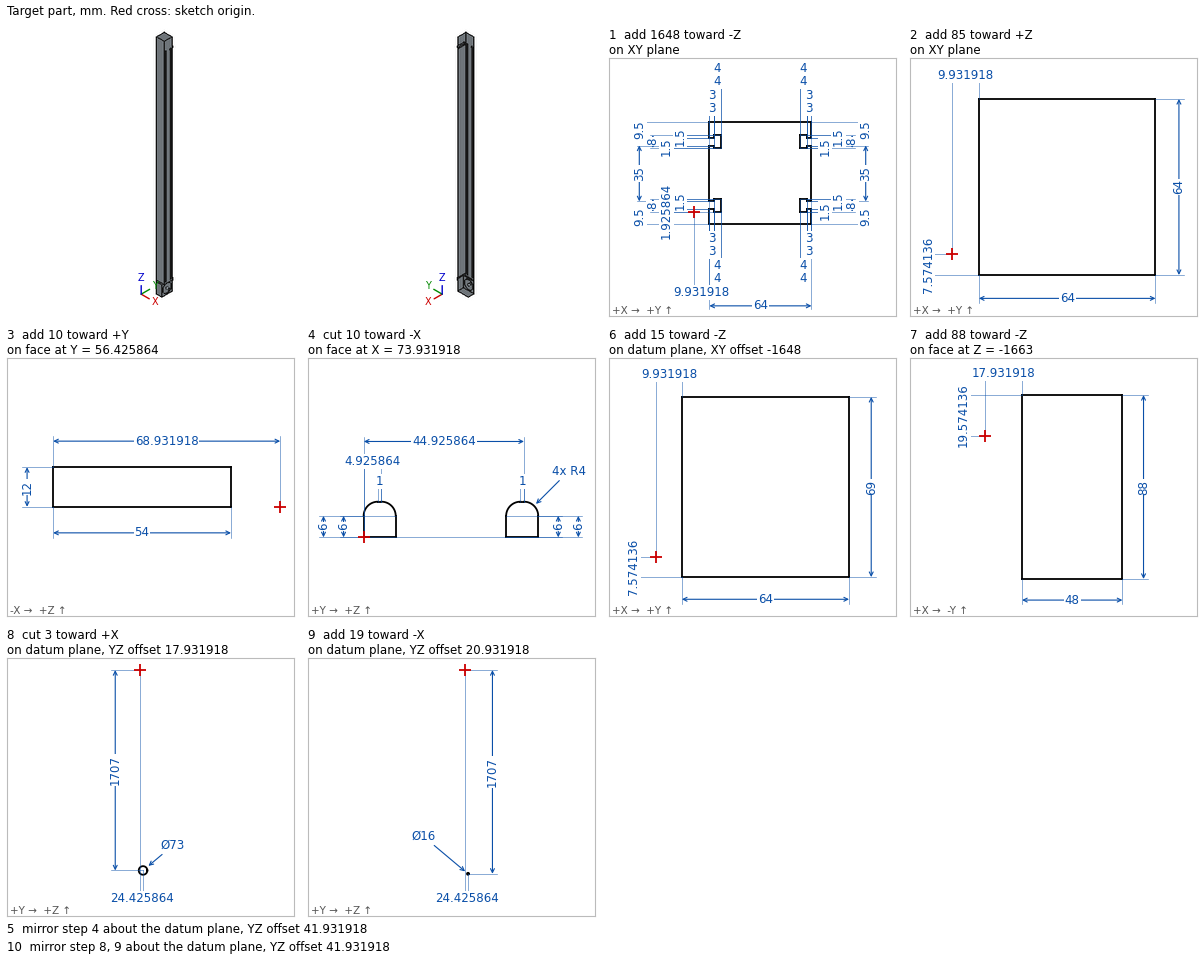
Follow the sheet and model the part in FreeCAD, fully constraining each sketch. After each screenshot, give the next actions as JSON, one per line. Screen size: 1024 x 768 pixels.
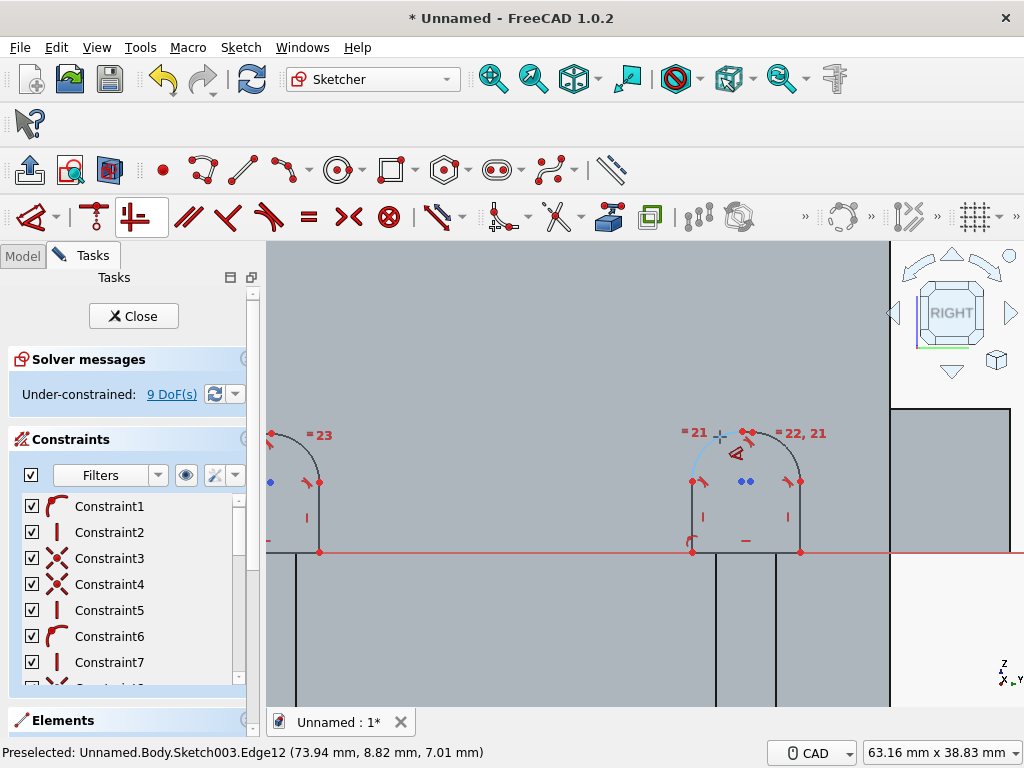
{"action": "left_click", "coordinate": [720, 437]}
{"action": "left_click", "coordinate": [706, 408]}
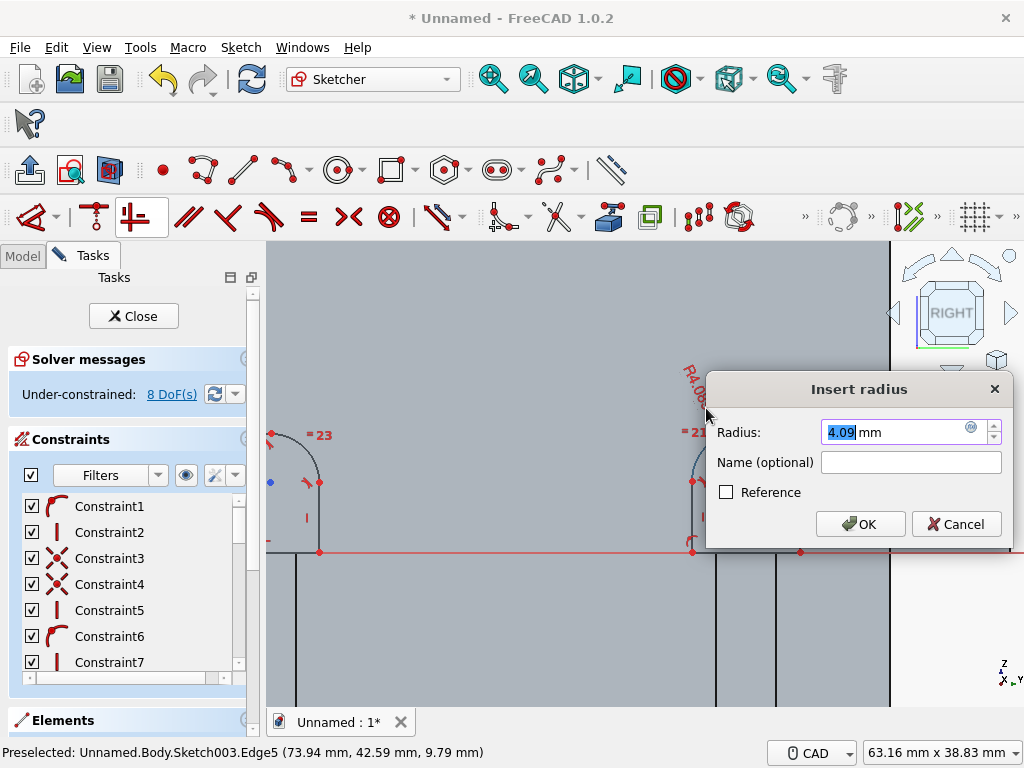
{"action": "type", "text": "4"}
{"action": "key", "text": "Return"}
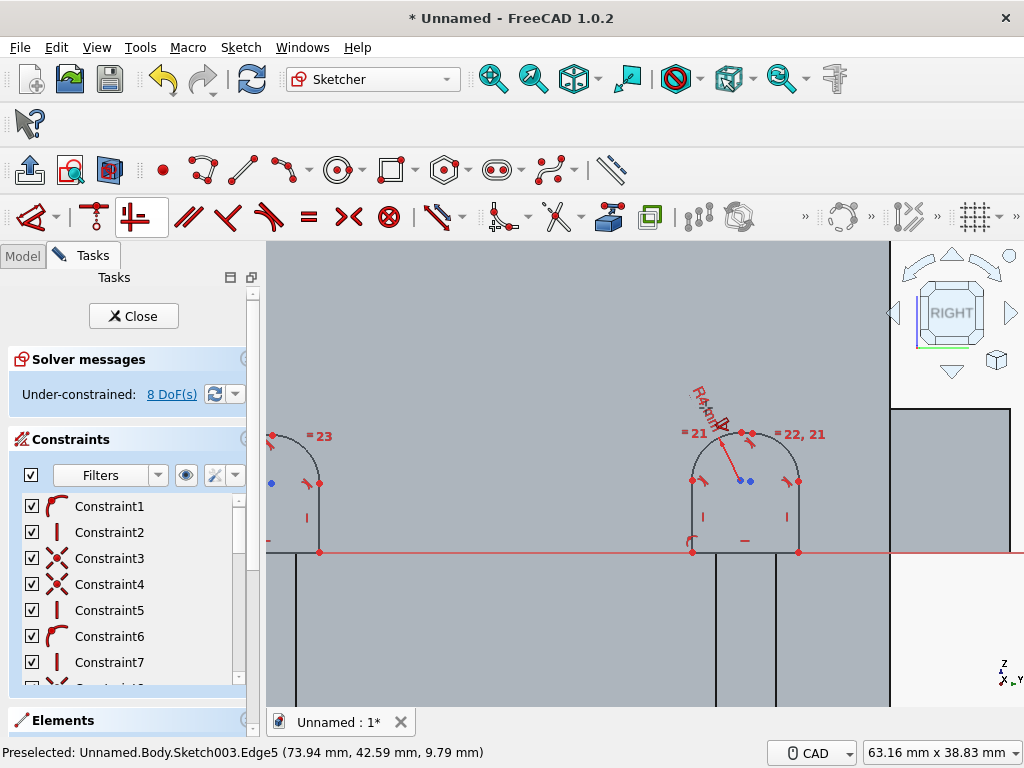
{"action": "scroll", "coordinate": [747, 433], "scroll_direction": "up", "scroll_amount": 6}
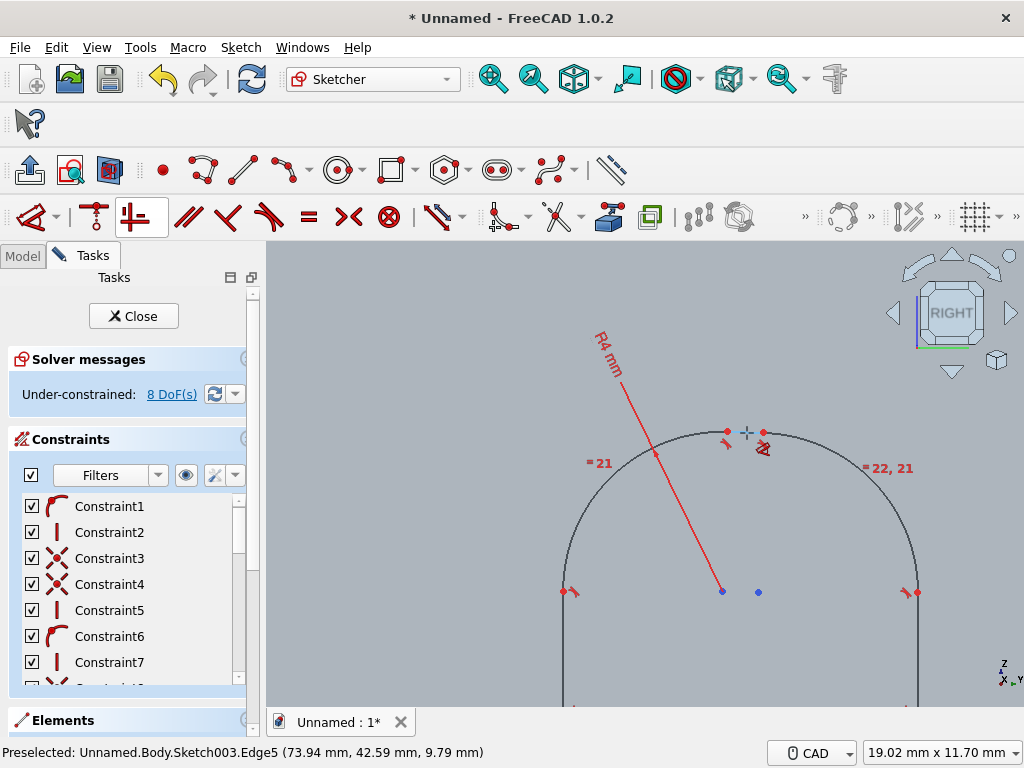
{"action": "left_click", "coordinate": [745, 432]}
{"action": "left_click", "coordinate": [745, 398]}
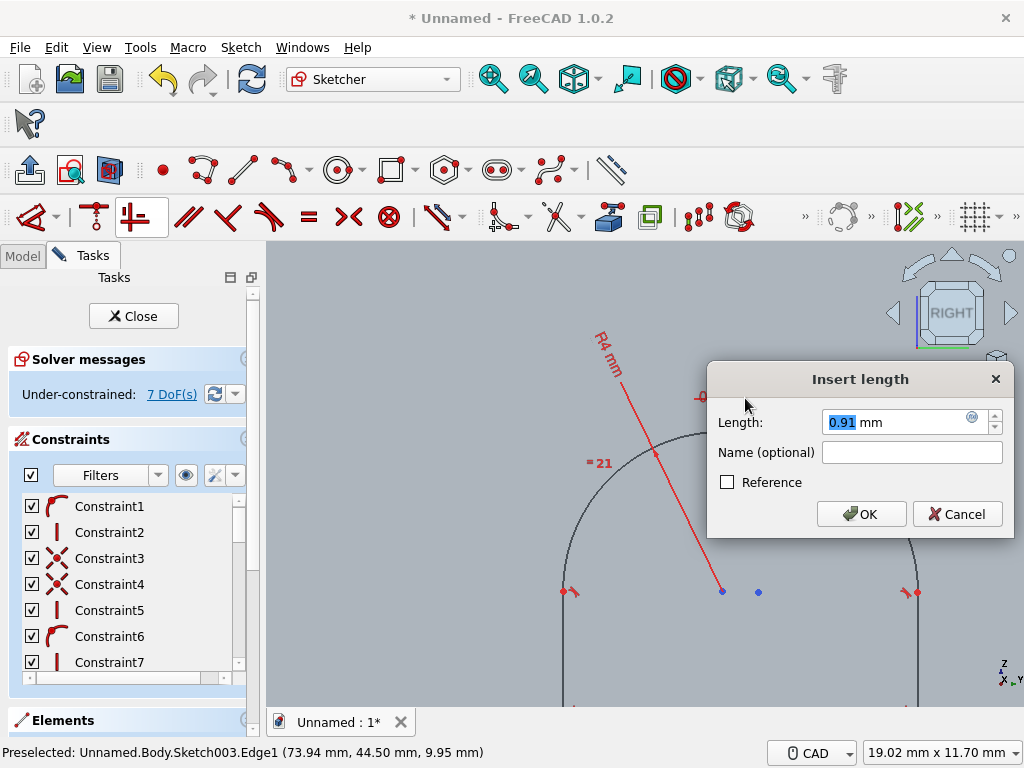
{"action": "type", "text": "1"}
{"action": "key", "text": "Return"}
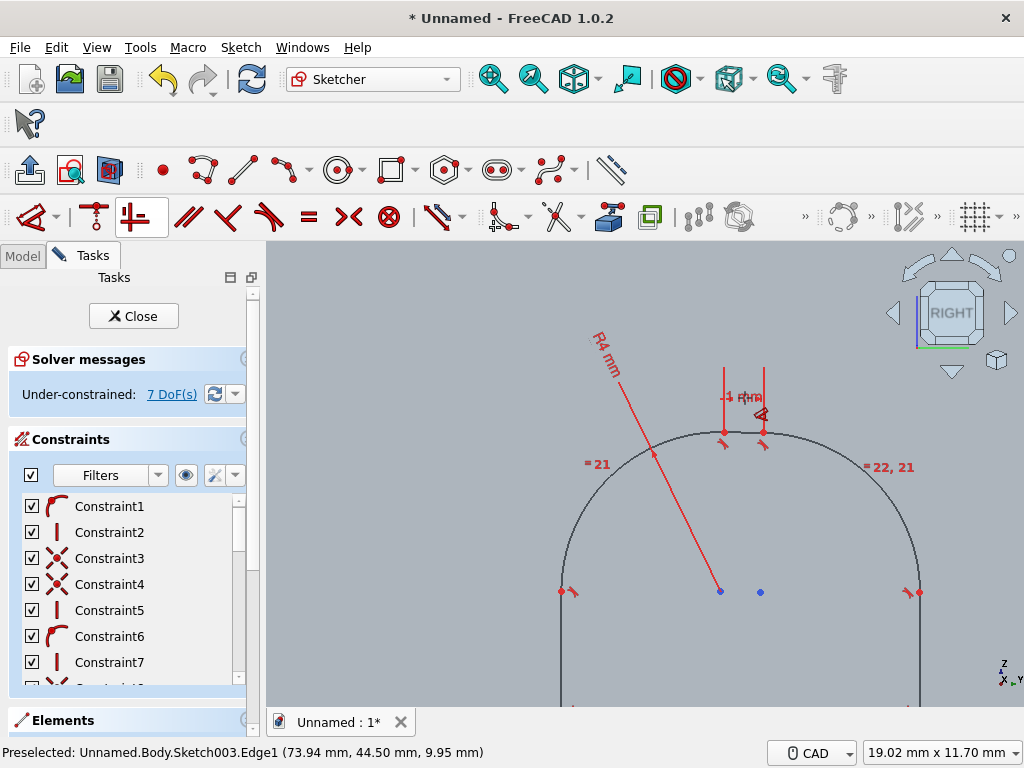
{"action": "scroll", "coordinate": [736, 435], "scroll_direction": "down", "scroll_amount": 8}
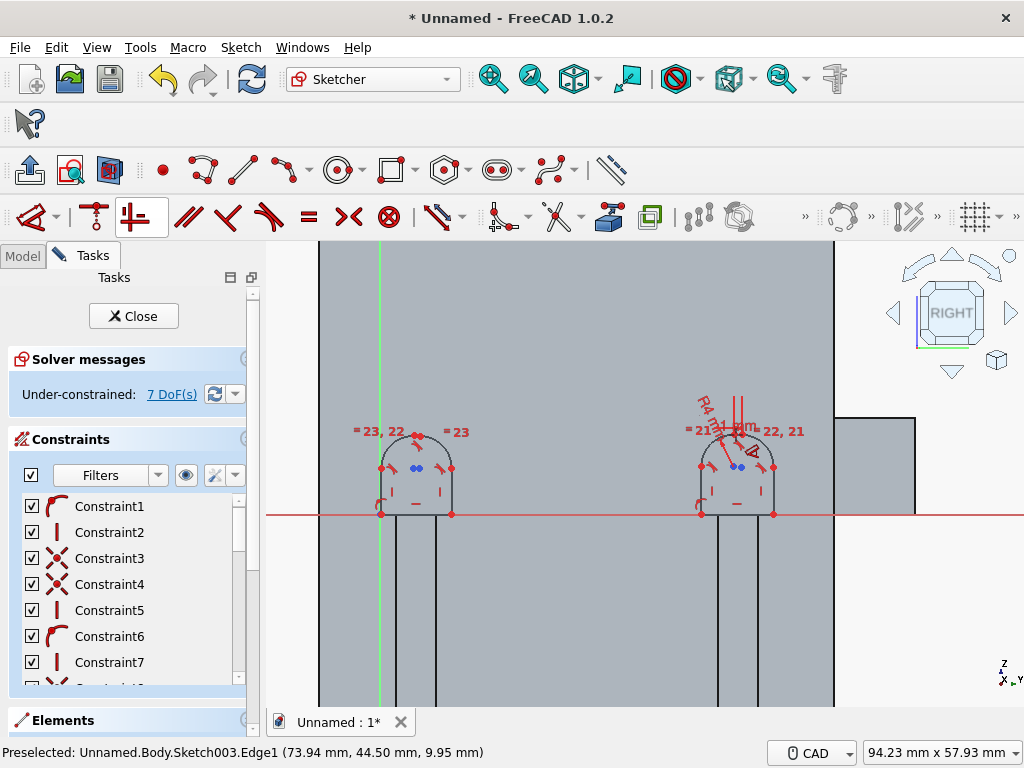
{"action": "left_click", "coordinate": [701, 481]}
{"action": "left_click", "coordinate": [735, 491]}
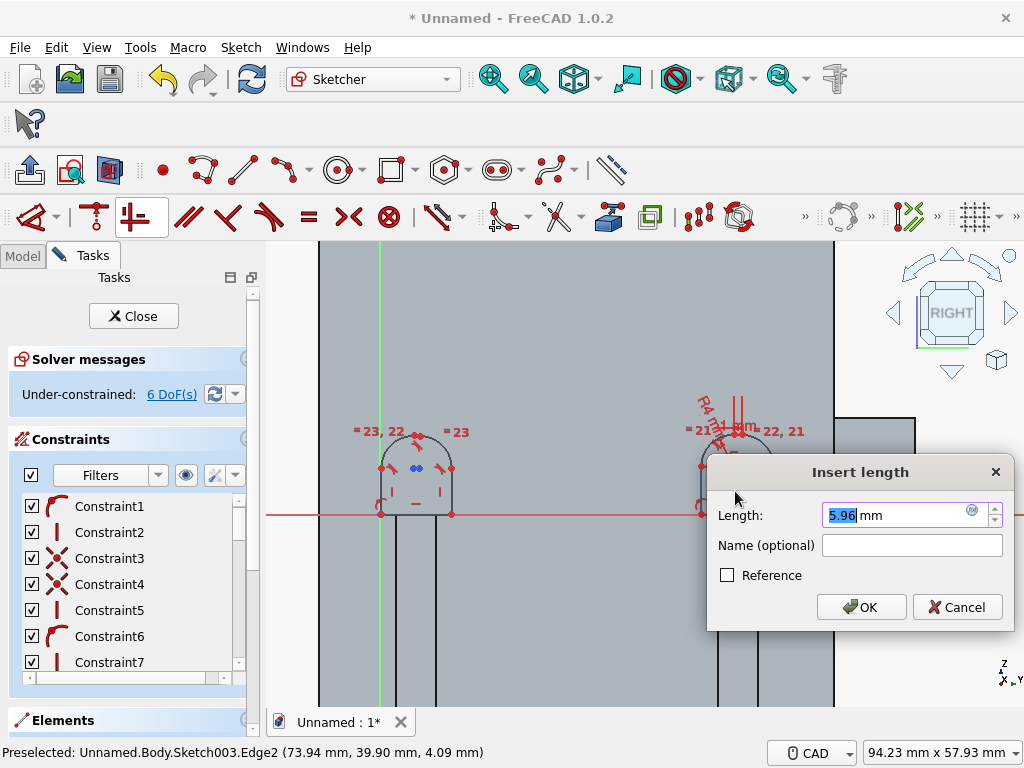
{"action": "type", "text": "6"}
{"action": "key", "text": "Return"}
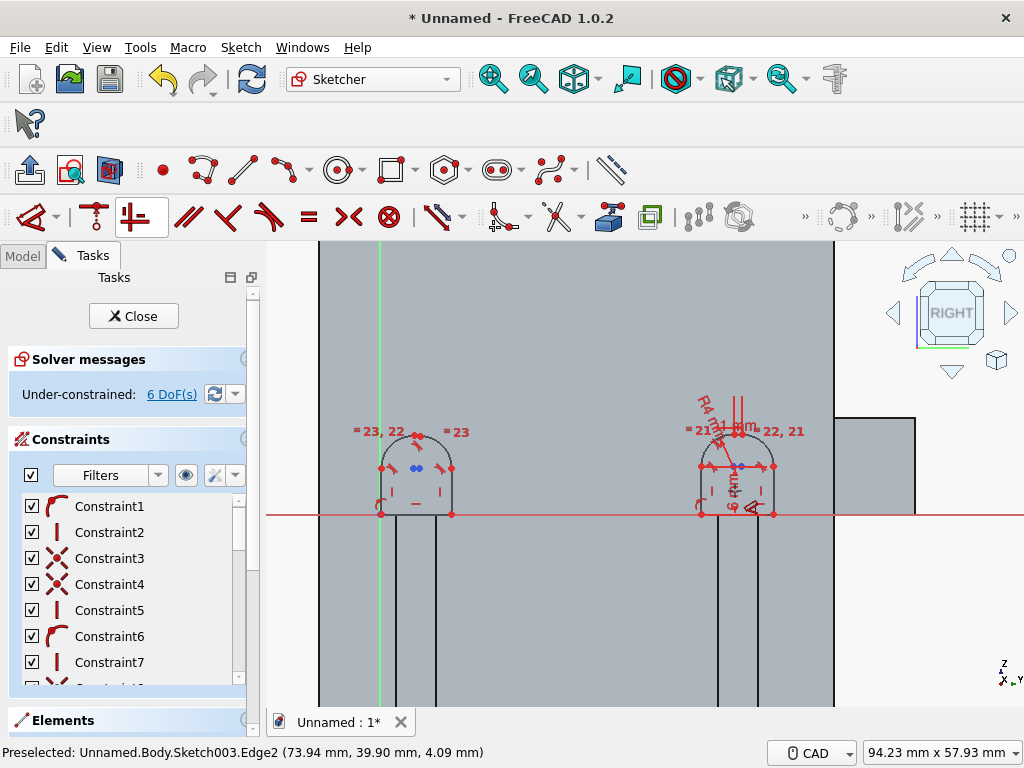
{"action": "scroll", "coordinate": [417, 436], "scroll_direction": "up", "scroll_amount": 8}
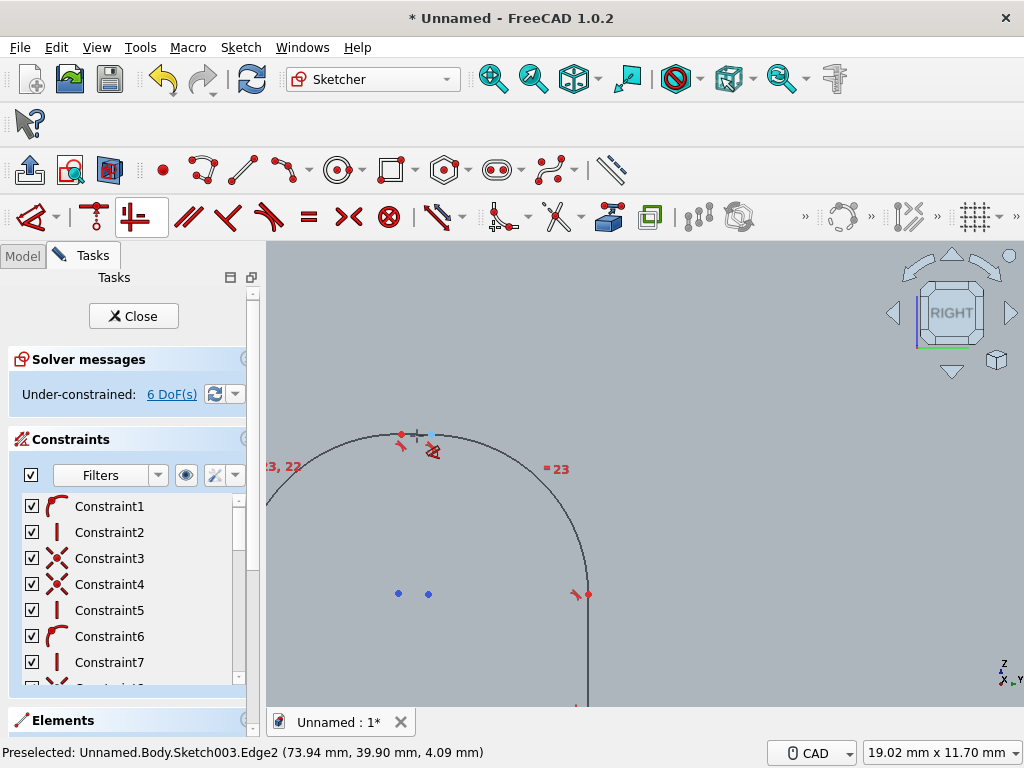
{"action": "left_click", "coordinate": [417, 435]}
{"action": "left_click", "coordinate": [417, 400]}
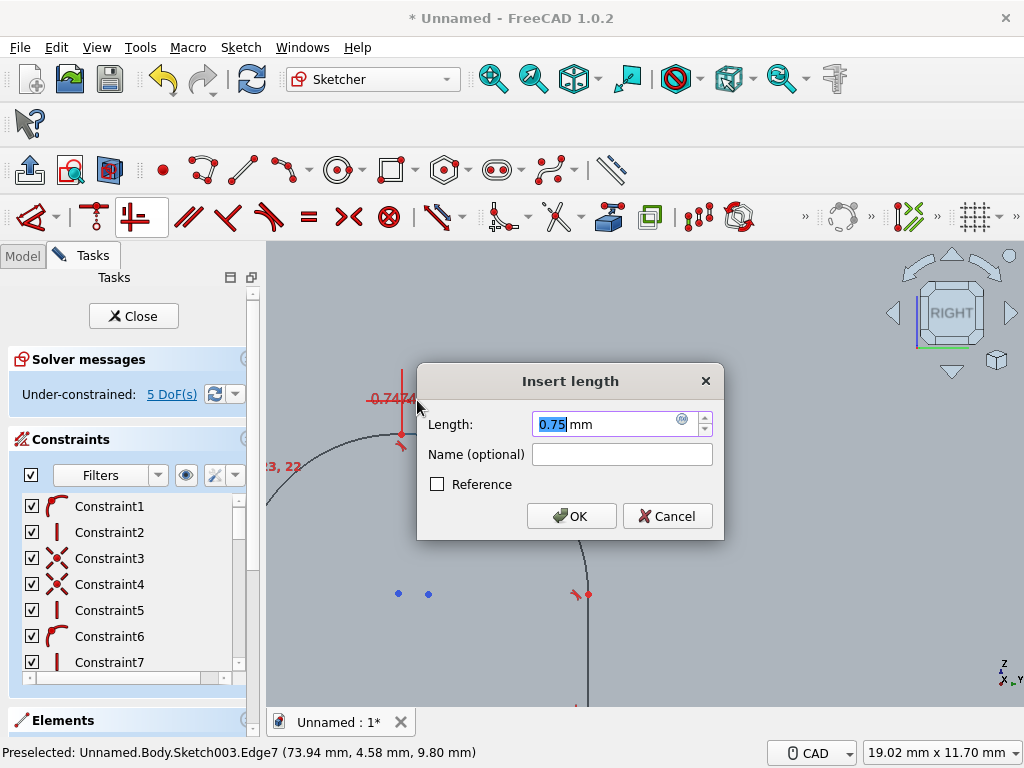
{"action": "type", "text": "1"}
{"action": "key", "text": "Return"}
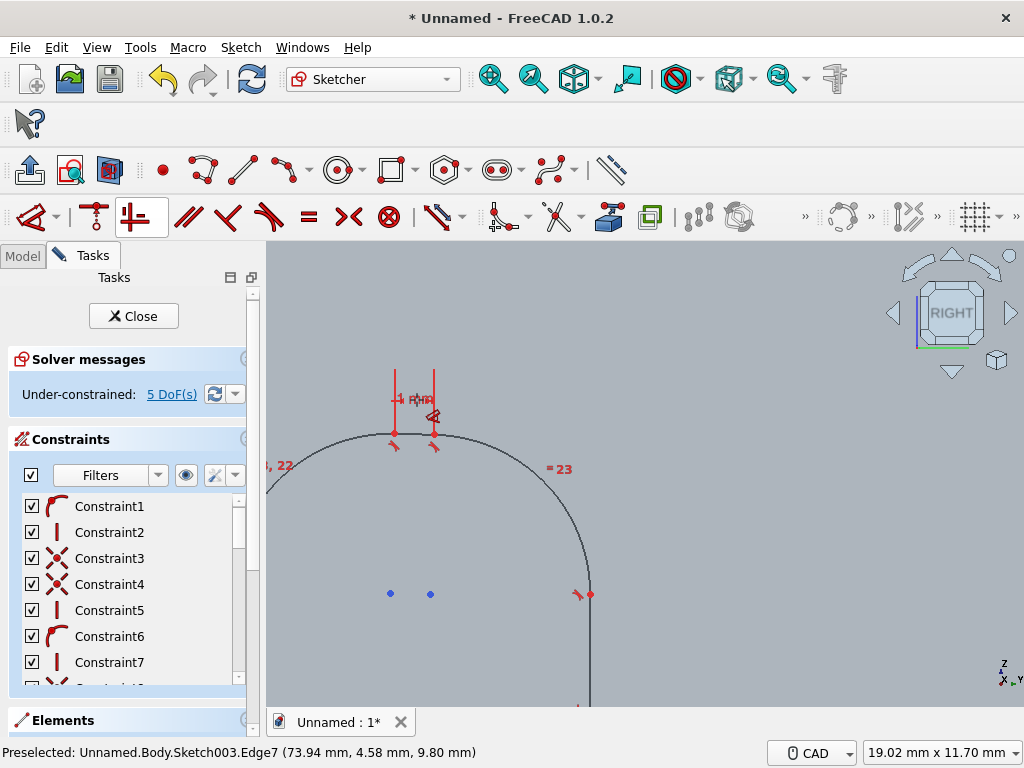
{"action": "scroll", "coordinate": [417, 436], "scroll_direction": "down", "scroll_amount": 8}